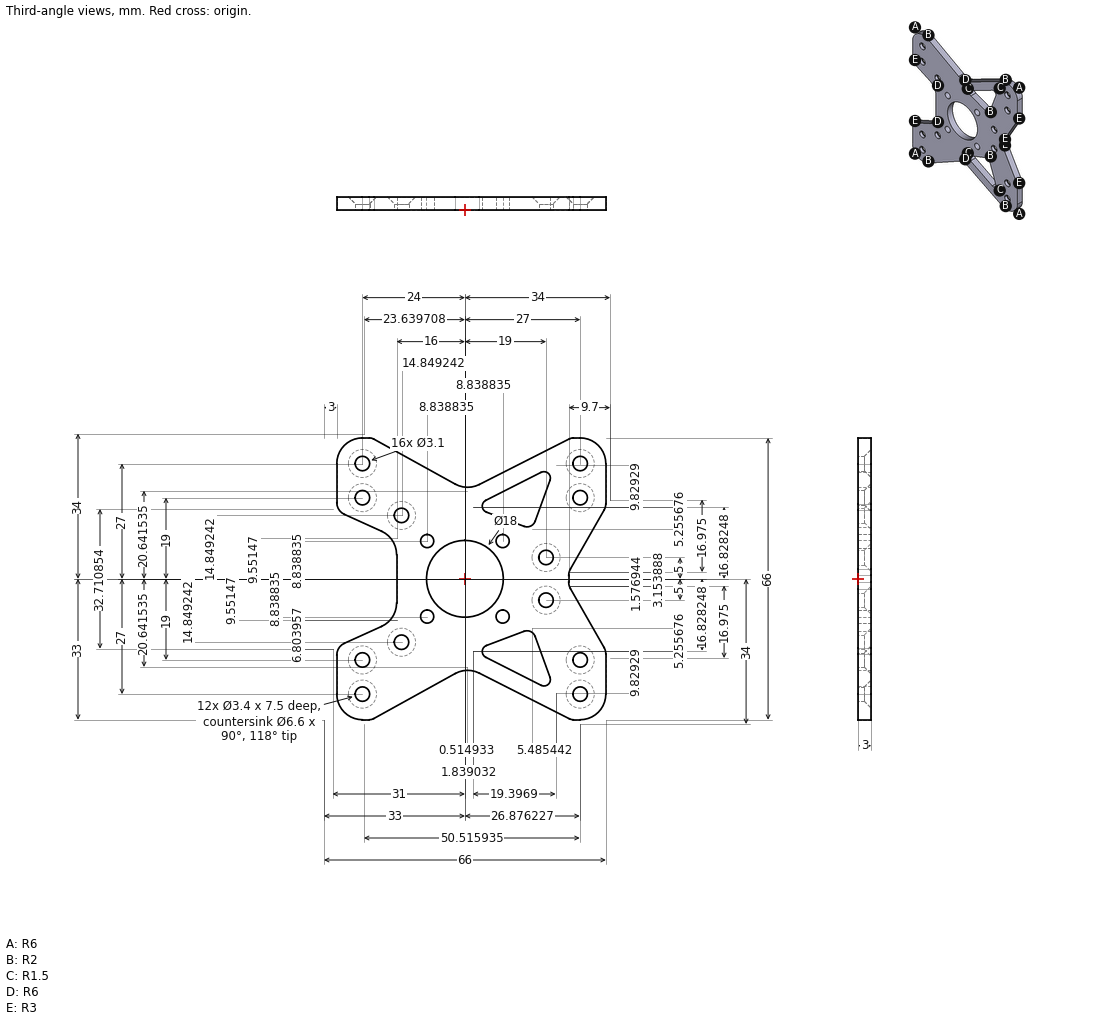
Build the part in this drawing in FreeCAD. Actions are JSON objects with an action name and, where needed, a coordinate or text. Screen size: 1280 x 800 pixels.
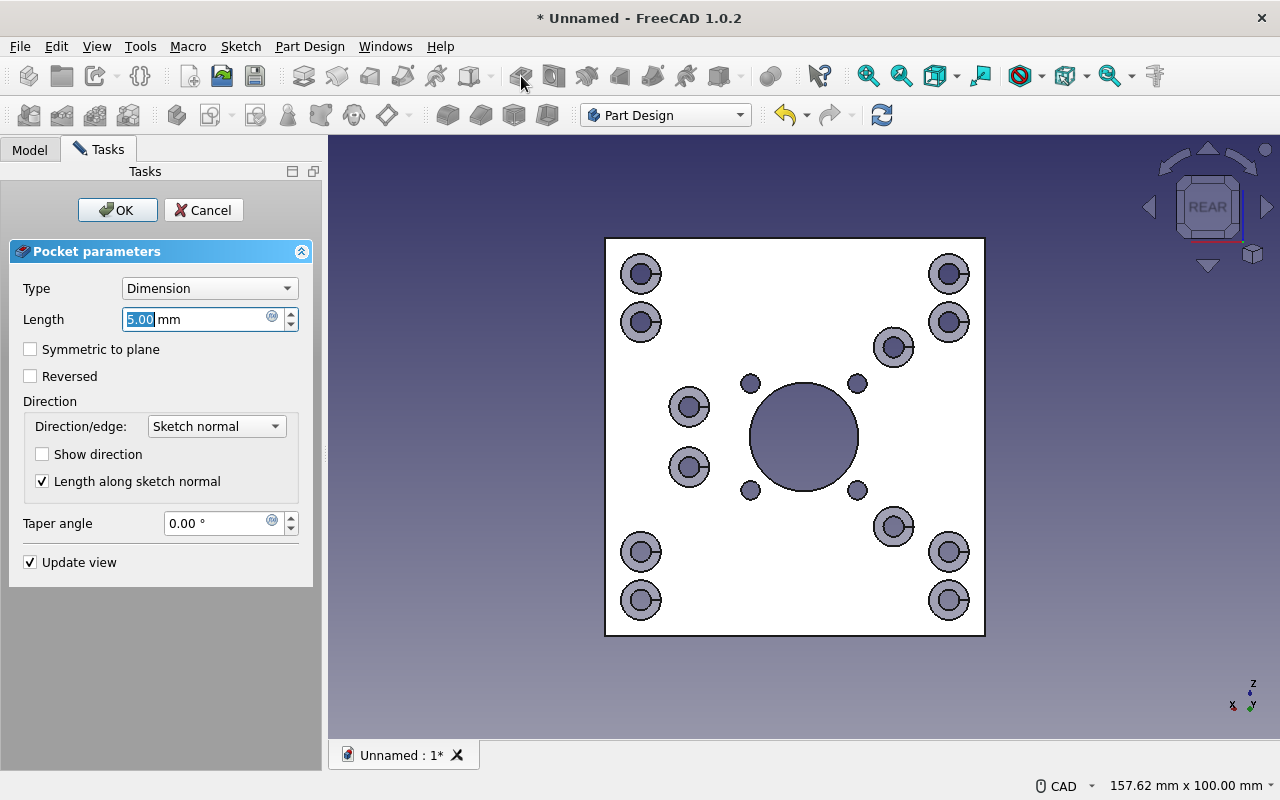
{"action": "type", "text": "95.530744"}
{"action": "key", "text": "Tab"}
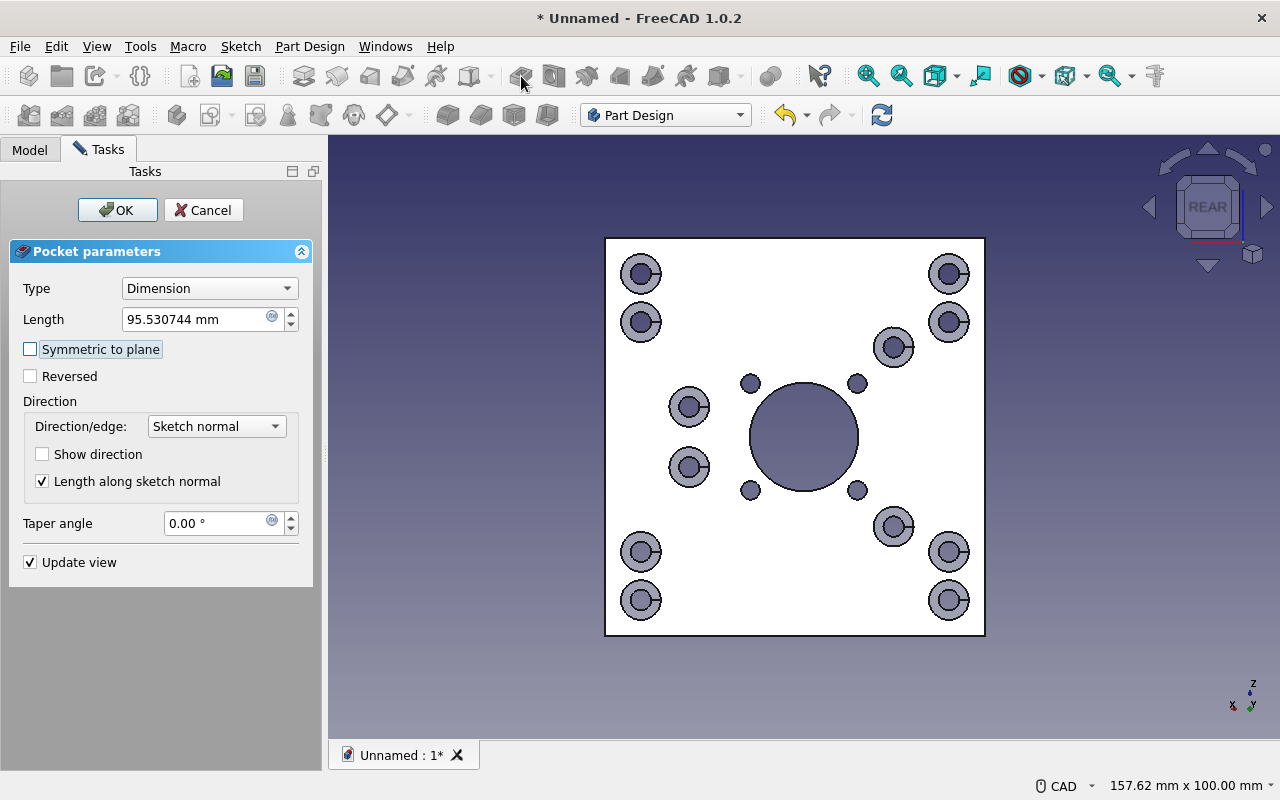
{"action": "left_click", "coordinate": [31, 349]}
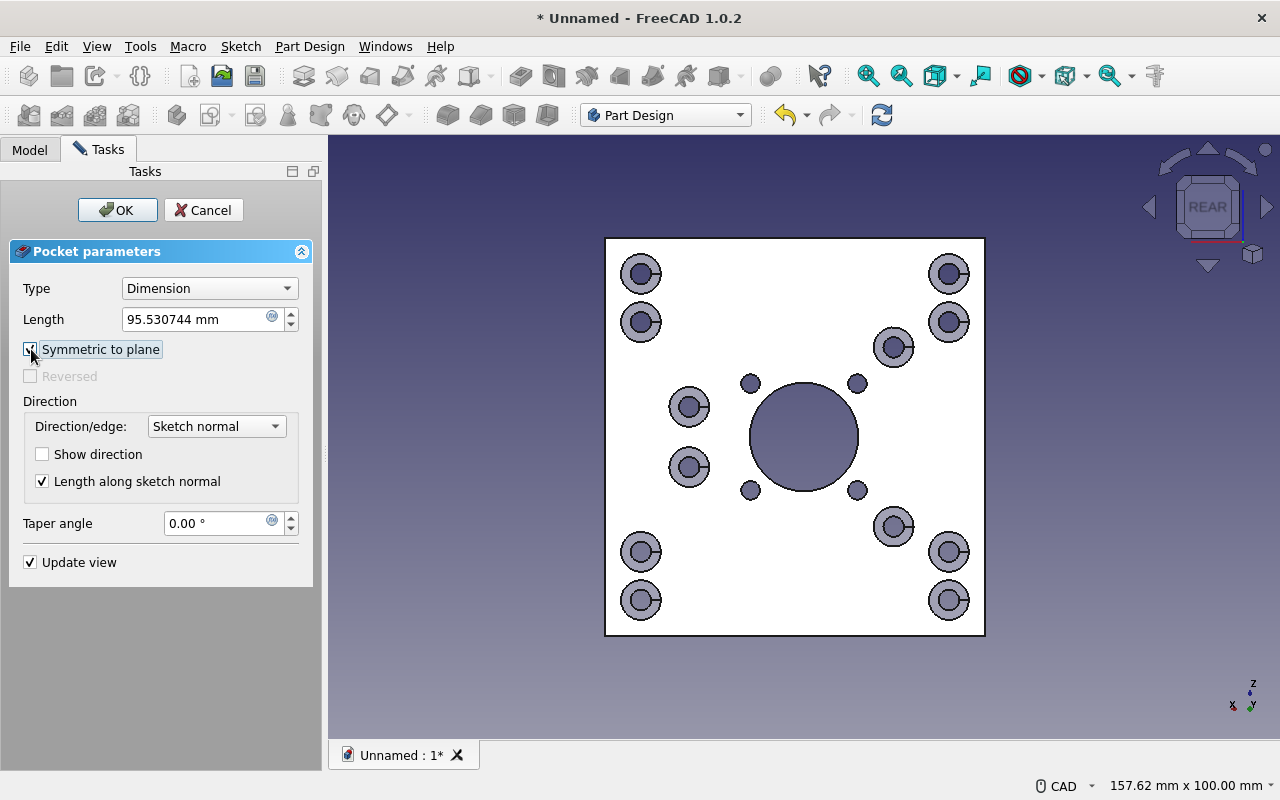
{"action": "left_click", "coordinate": [118, 210]}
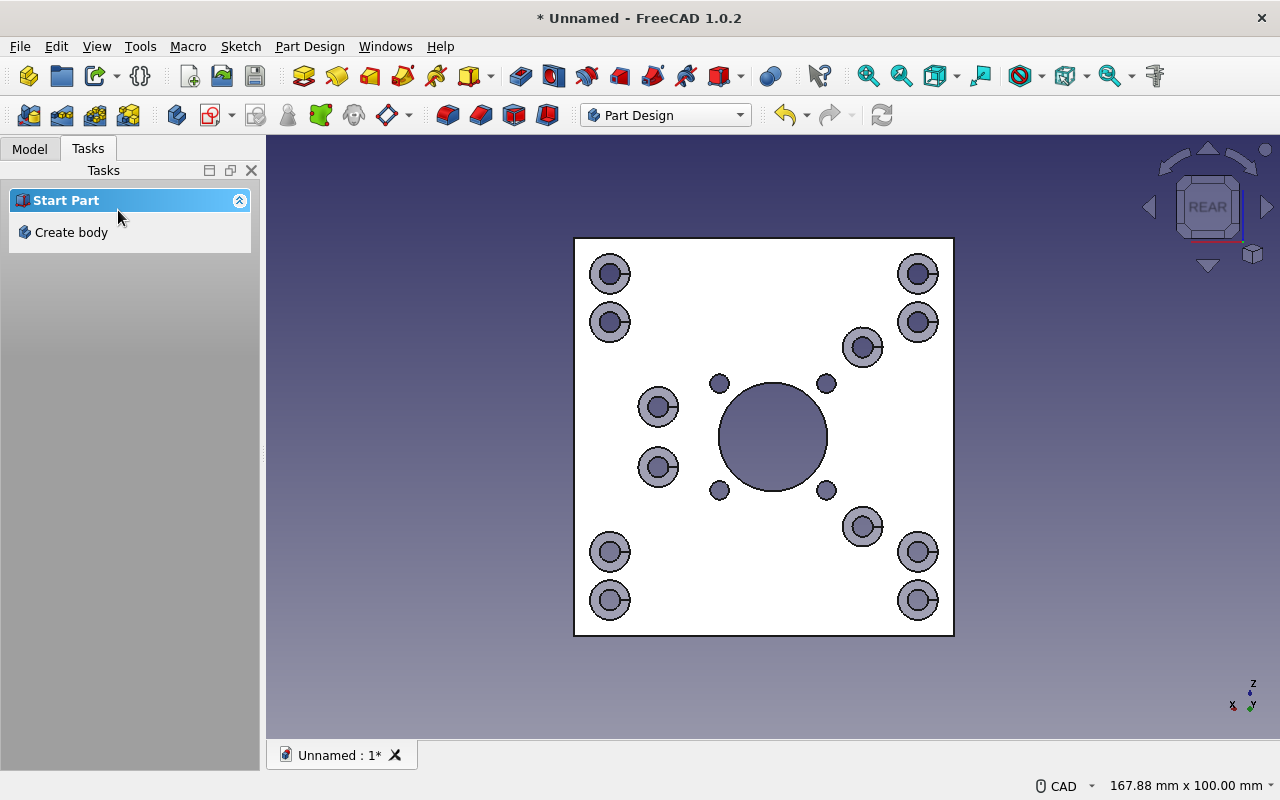
{"action": "scroll", "coordinate": [954, 635], "scroll_direction": "up", "scroll_amount": 4}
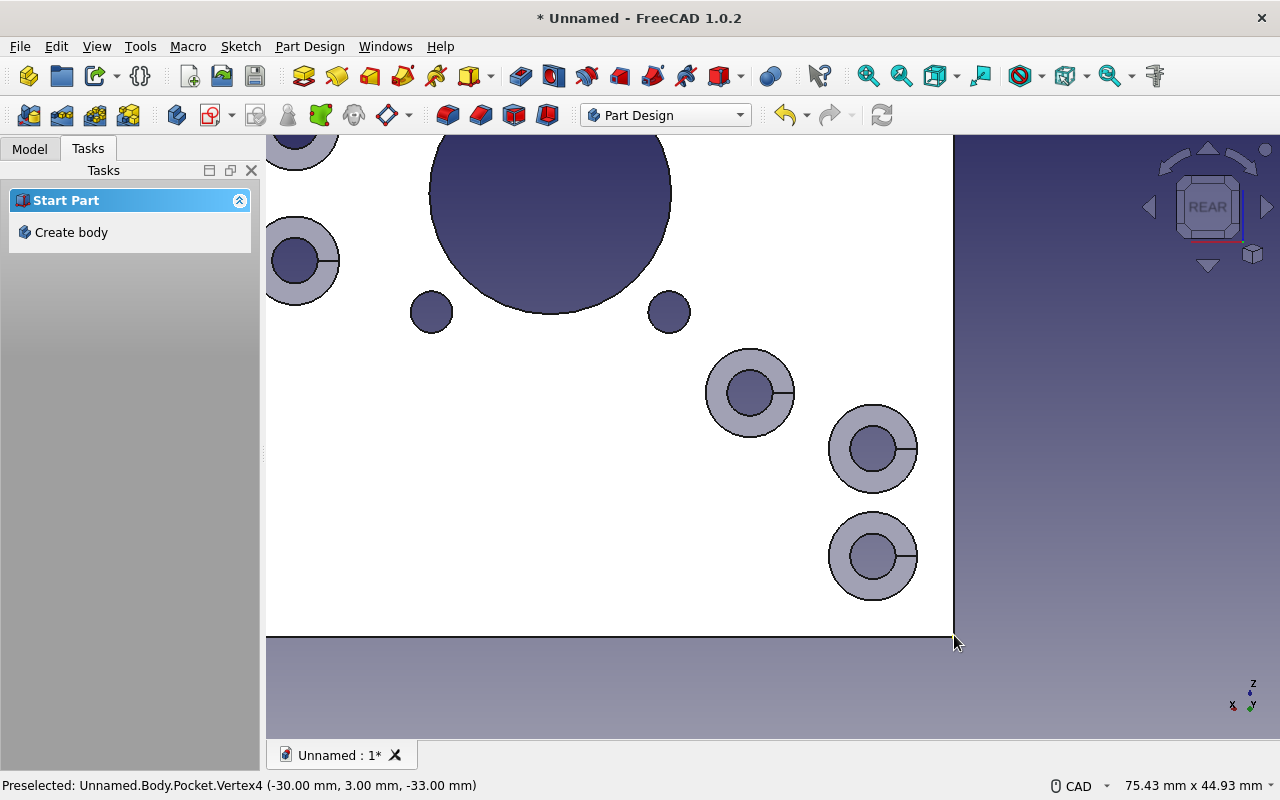
{"action": "left_click", "coordinate": [869, 76]}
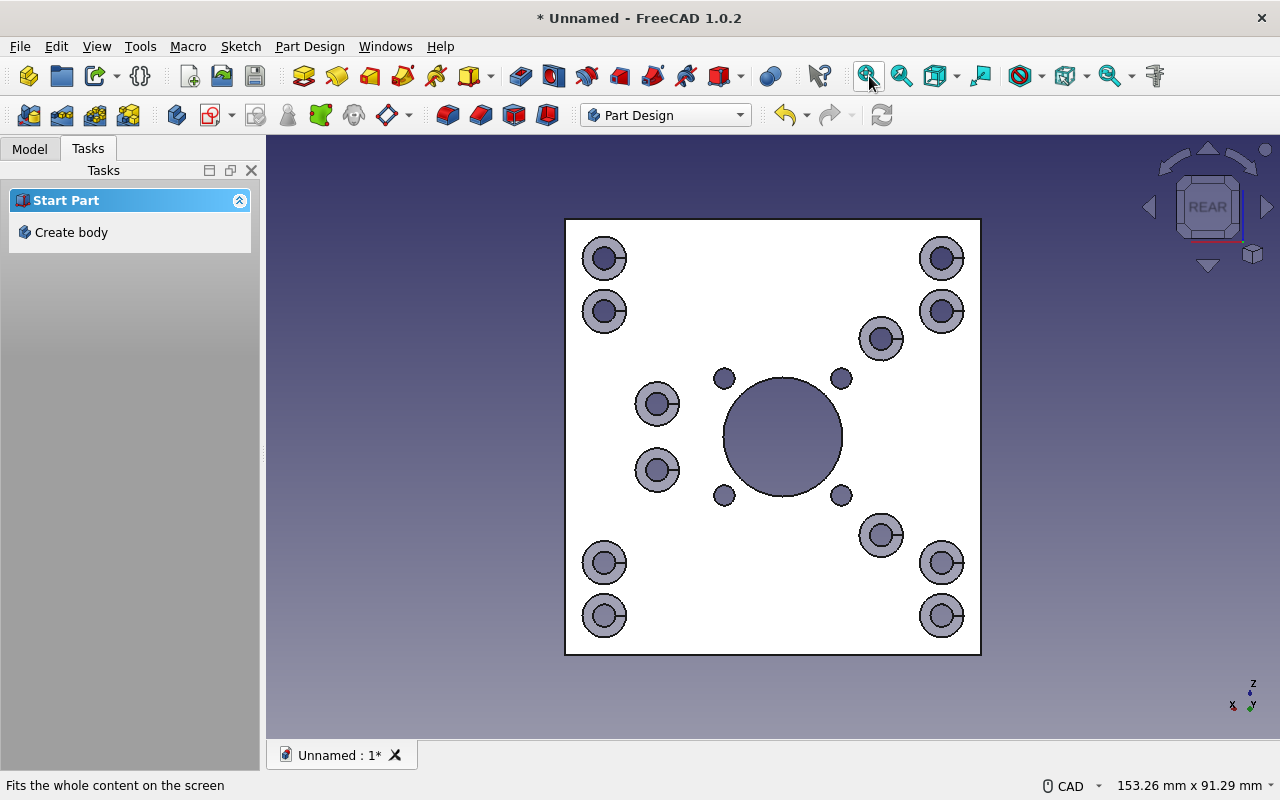
{"action": "key", "text": "0"}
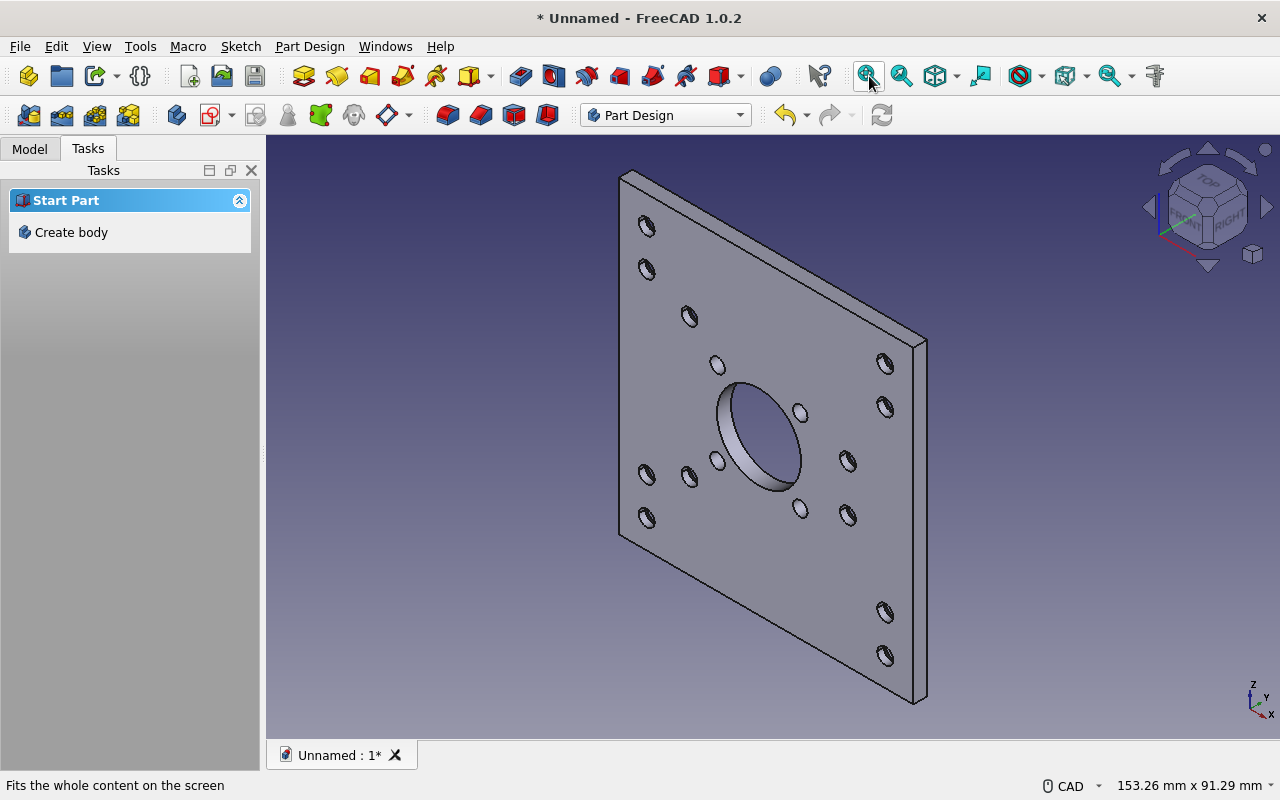
{"action": "left_click", "coordinate": [920, 343]}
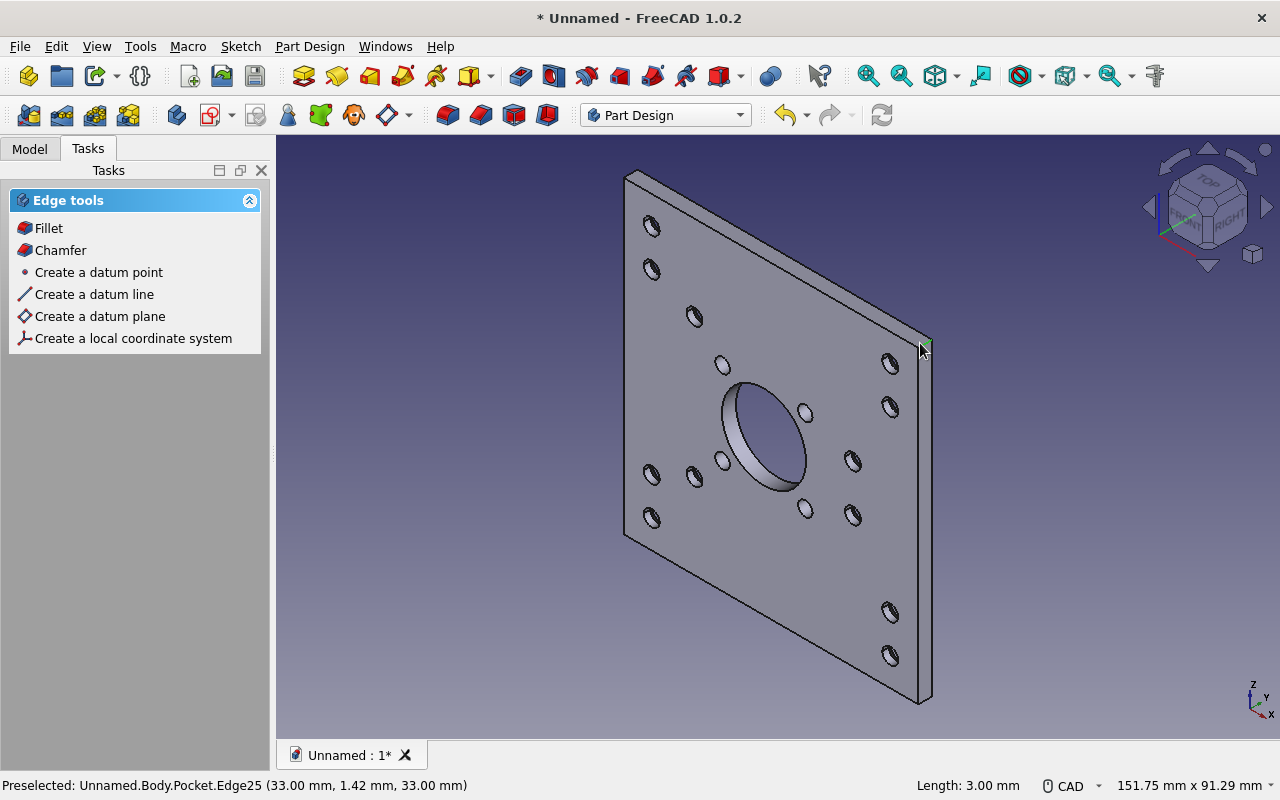
{"action": "scroll", "coordinate": [631, 529], "scroll_direction": "up", "scroll_amount": 4}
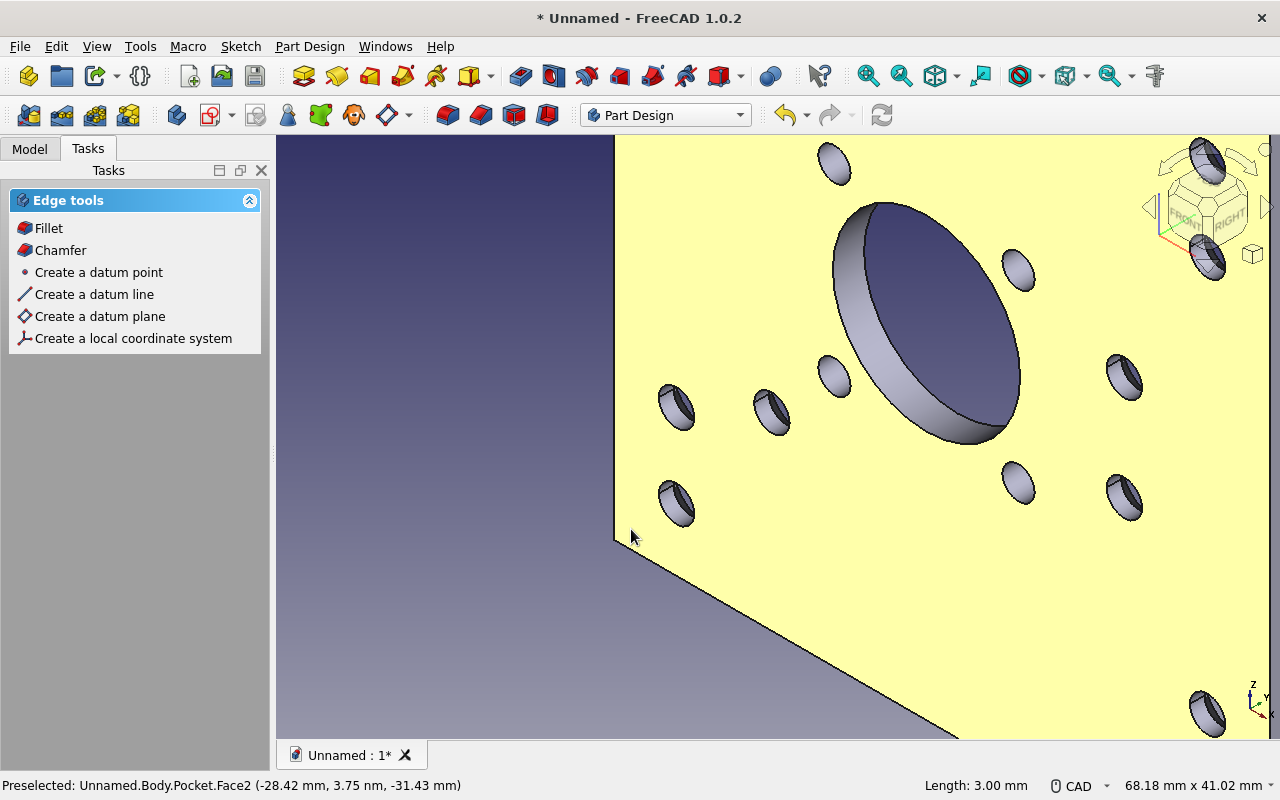
{"action": "left_click", "coordinate": [869, 76]}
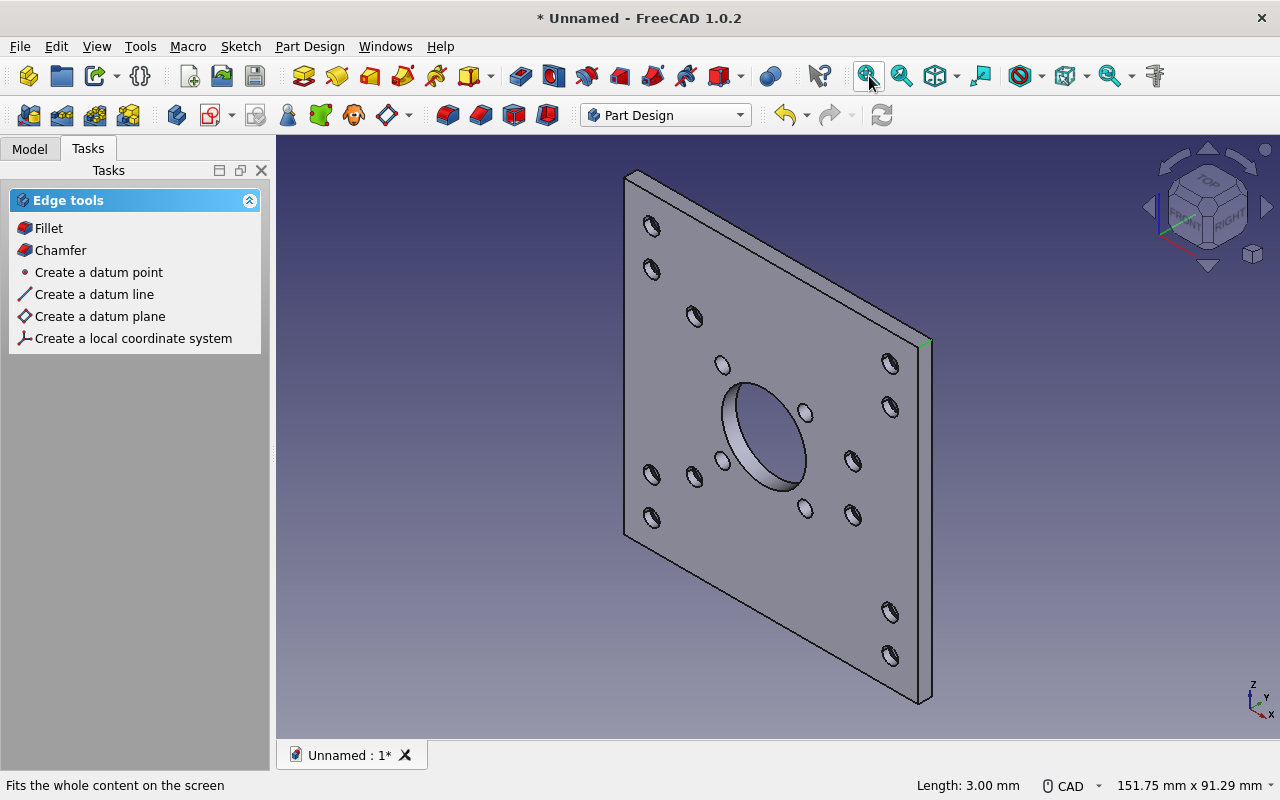
{"action": "key", "text": "2"}